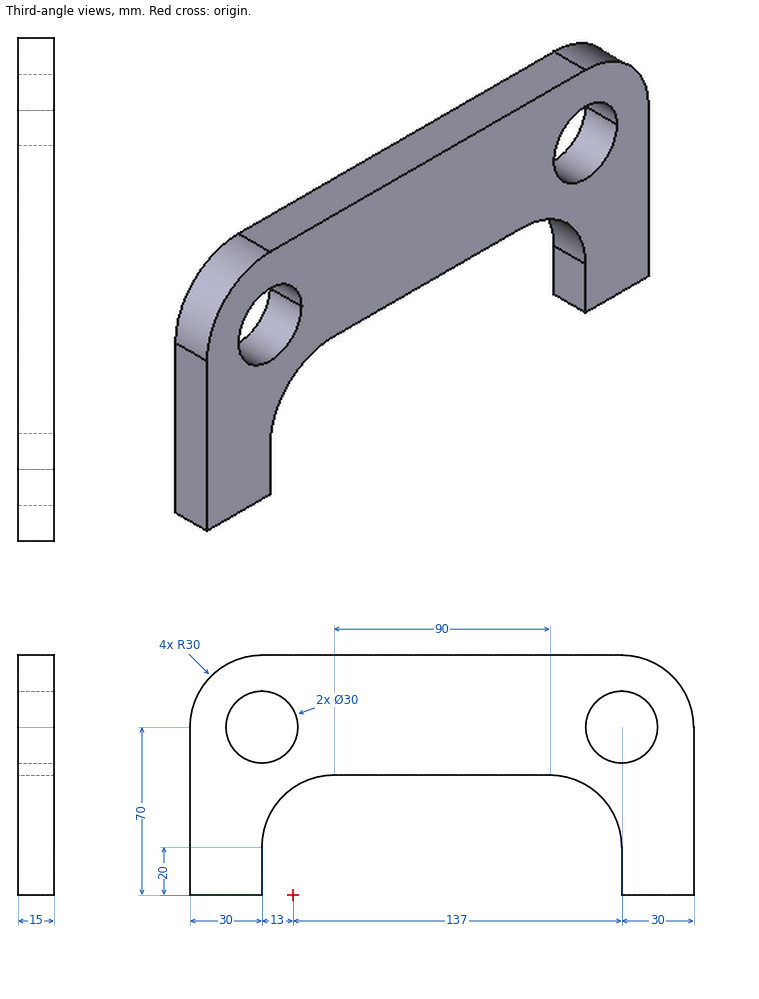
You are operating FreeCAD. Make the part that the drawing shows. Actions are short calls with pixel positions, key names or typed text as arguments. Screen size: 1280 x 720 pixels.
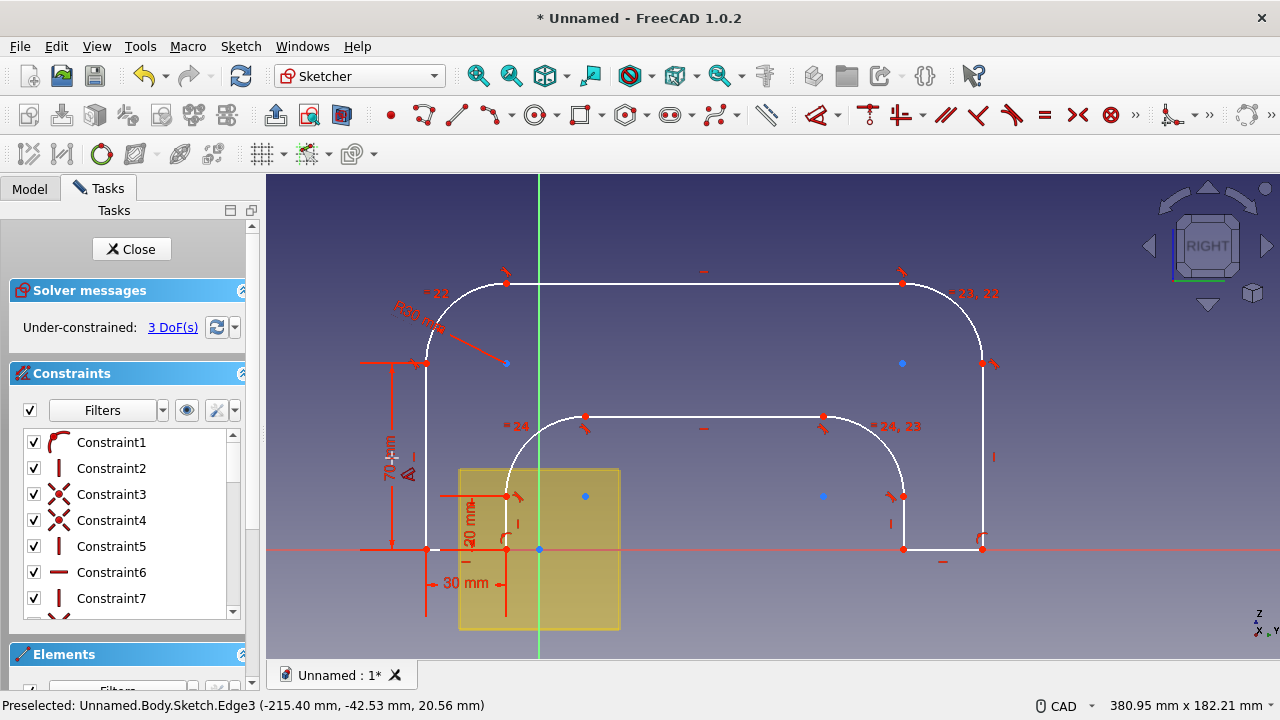
click(959, 550)
click(943, 584)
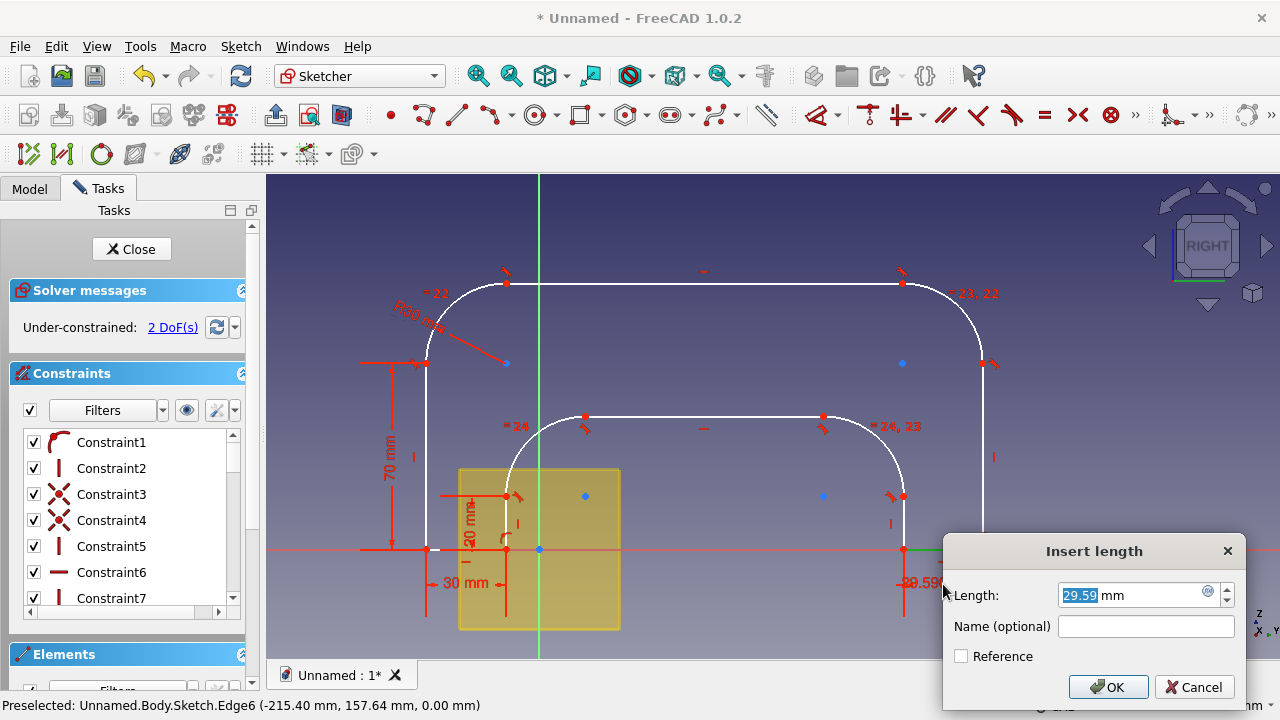
text(30)
key(Return)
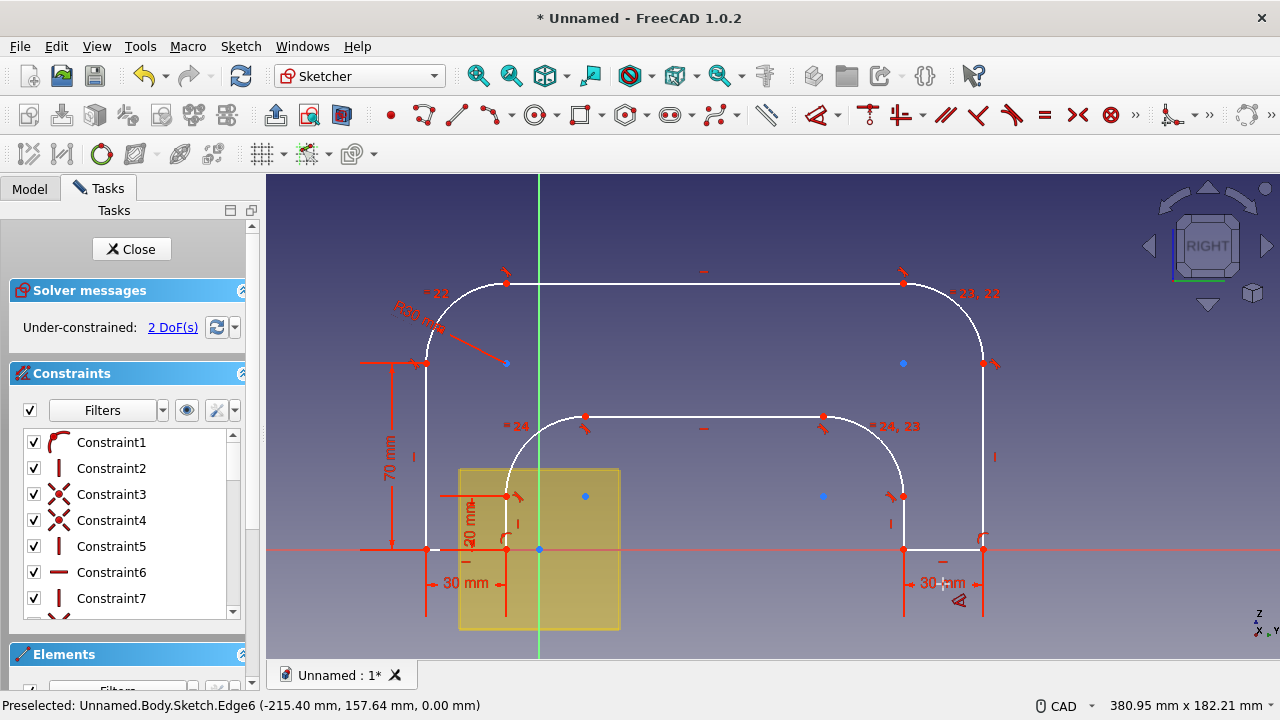
click(752, 417)
click(705, 451)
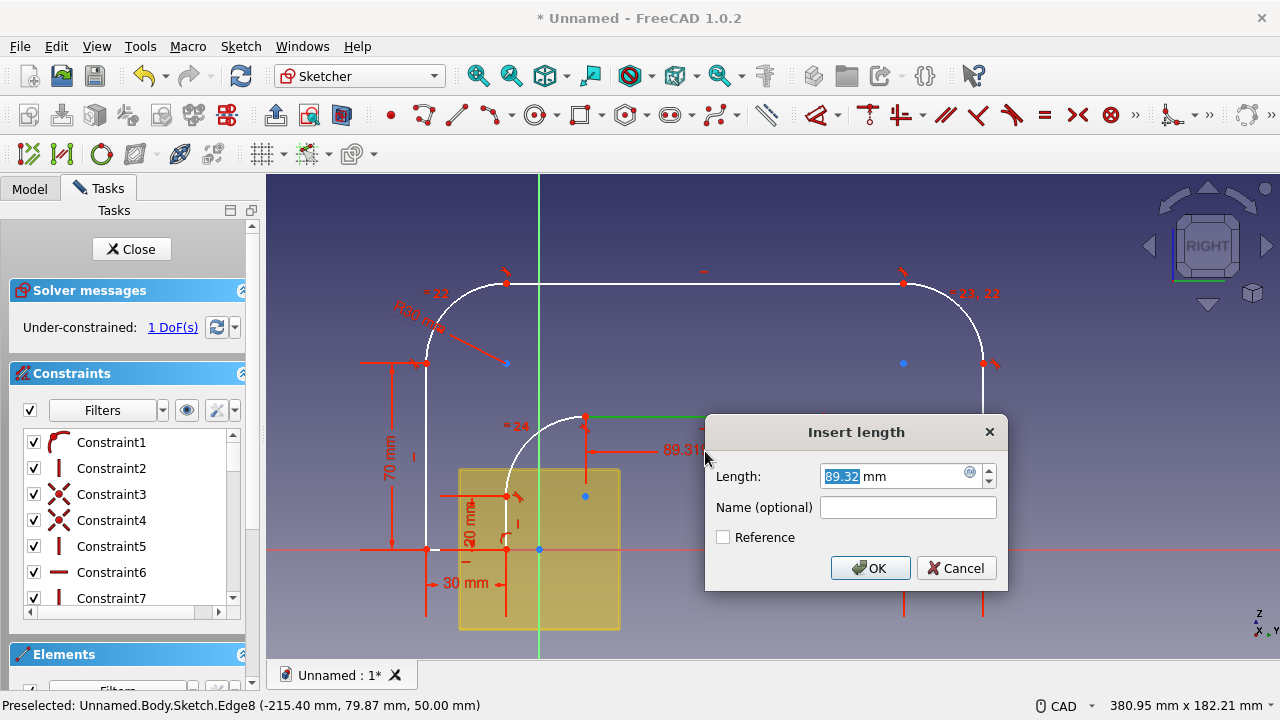
text(90)
key(Return)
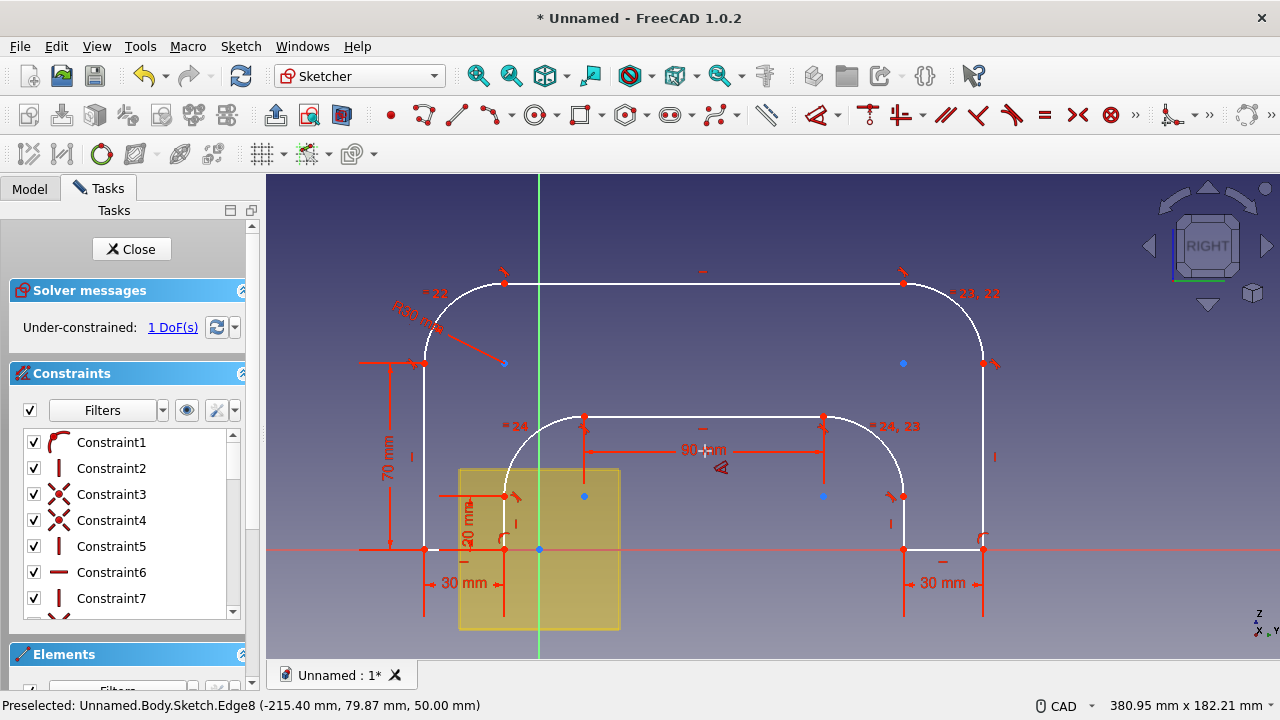
click(504, 496)
click(522, 608)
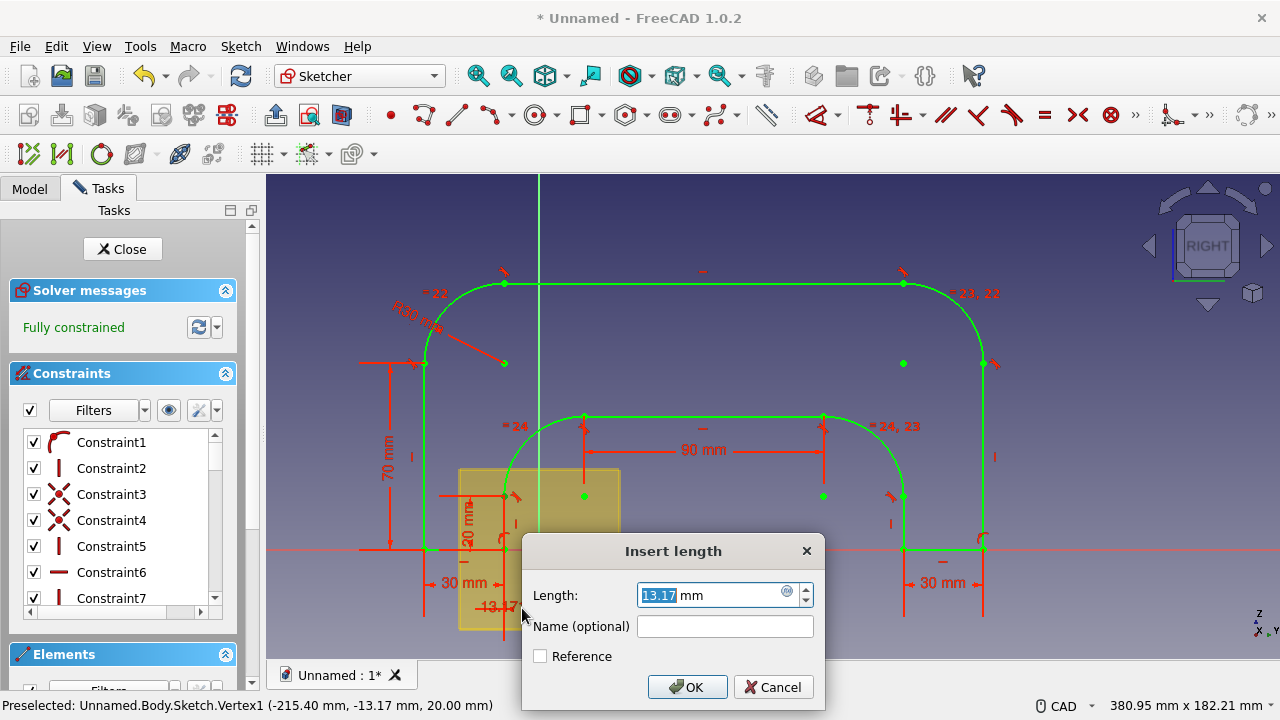
text(13)
key(Return)
key(Escape)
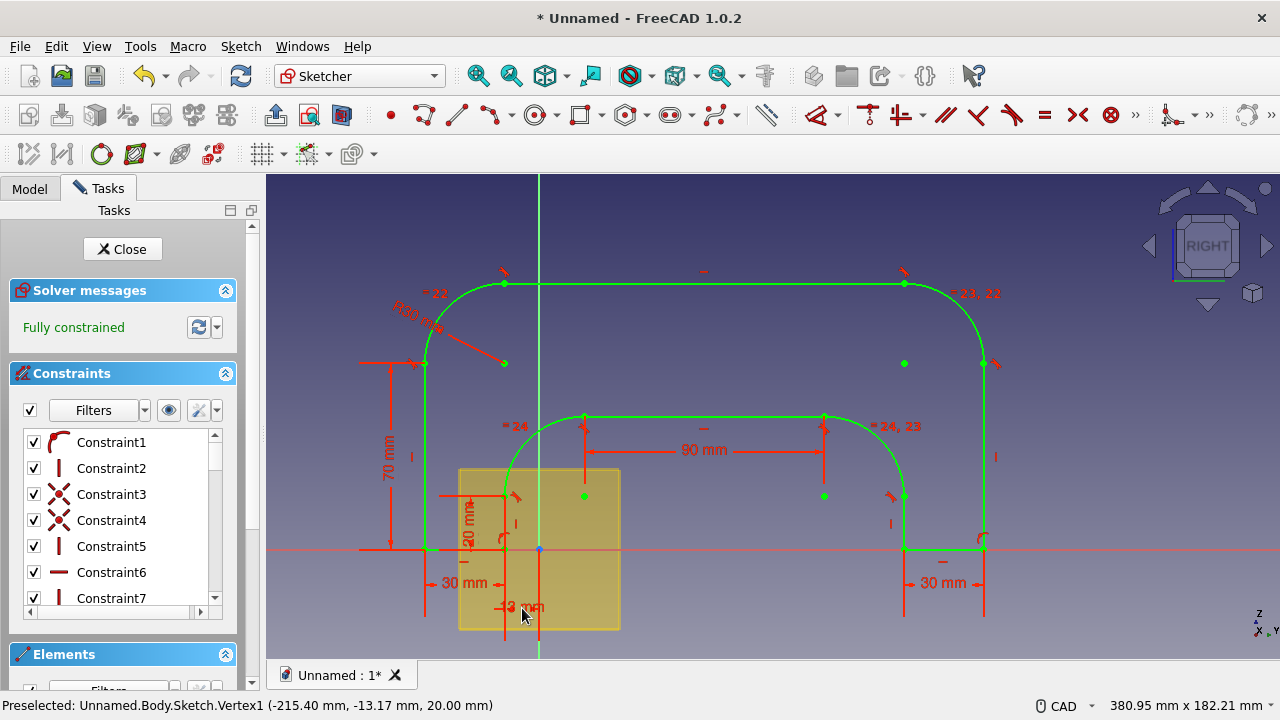
click(123, 249)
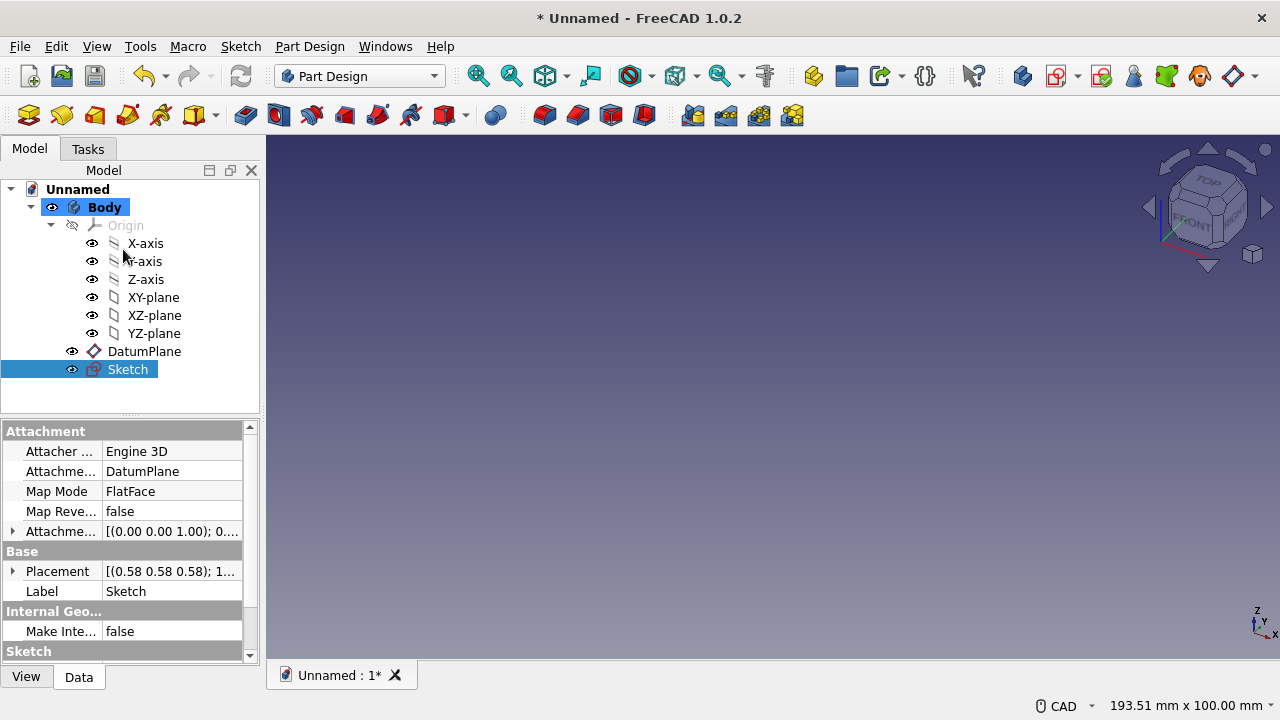
click(29, 116)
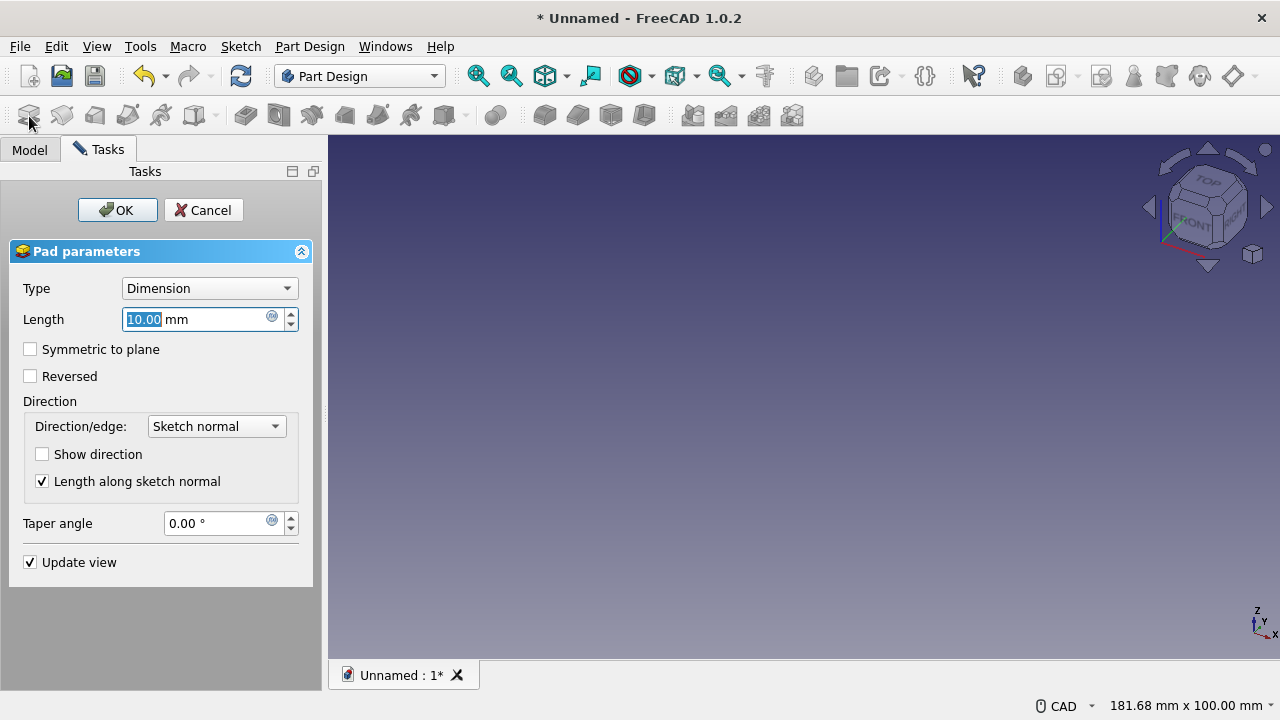
text(15)
key(Tab)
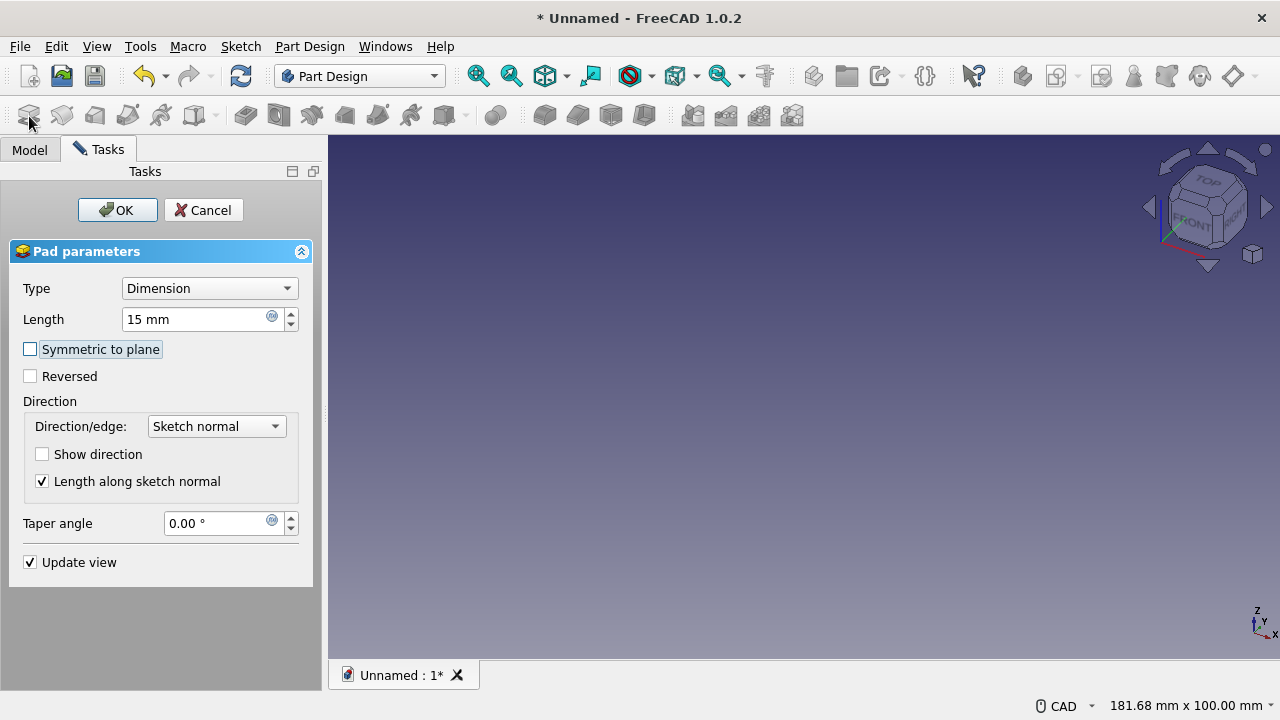
click(31, 376)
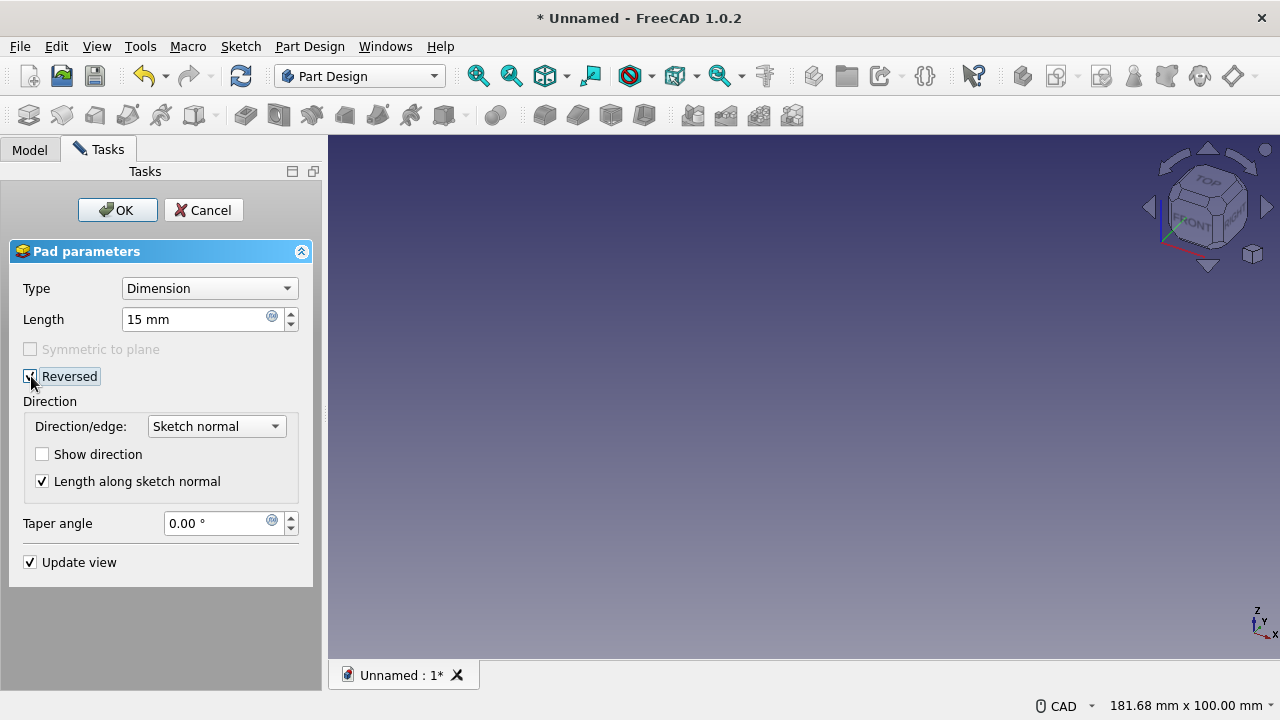
click(118, 210)